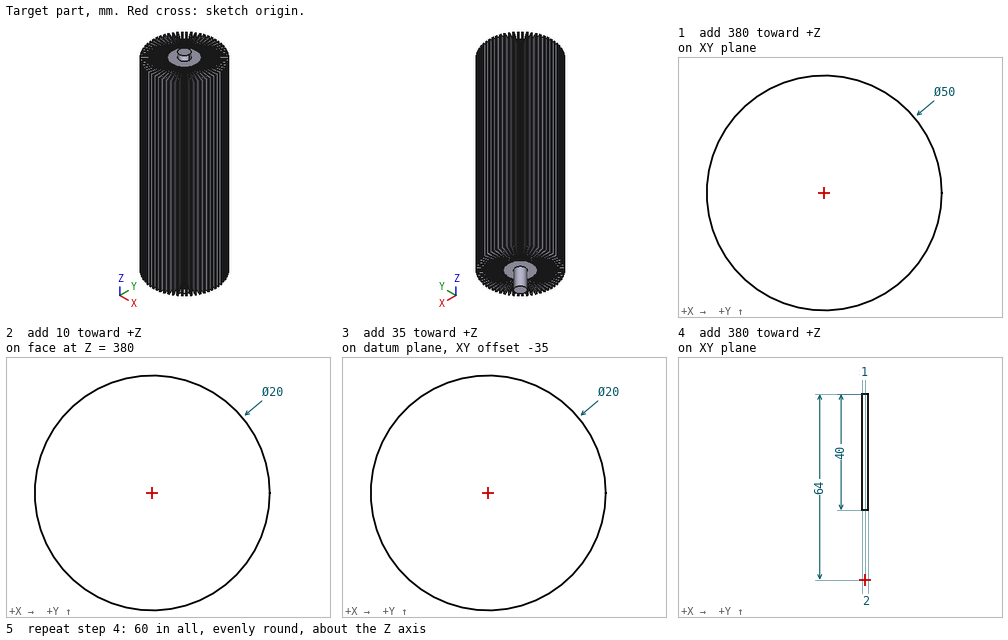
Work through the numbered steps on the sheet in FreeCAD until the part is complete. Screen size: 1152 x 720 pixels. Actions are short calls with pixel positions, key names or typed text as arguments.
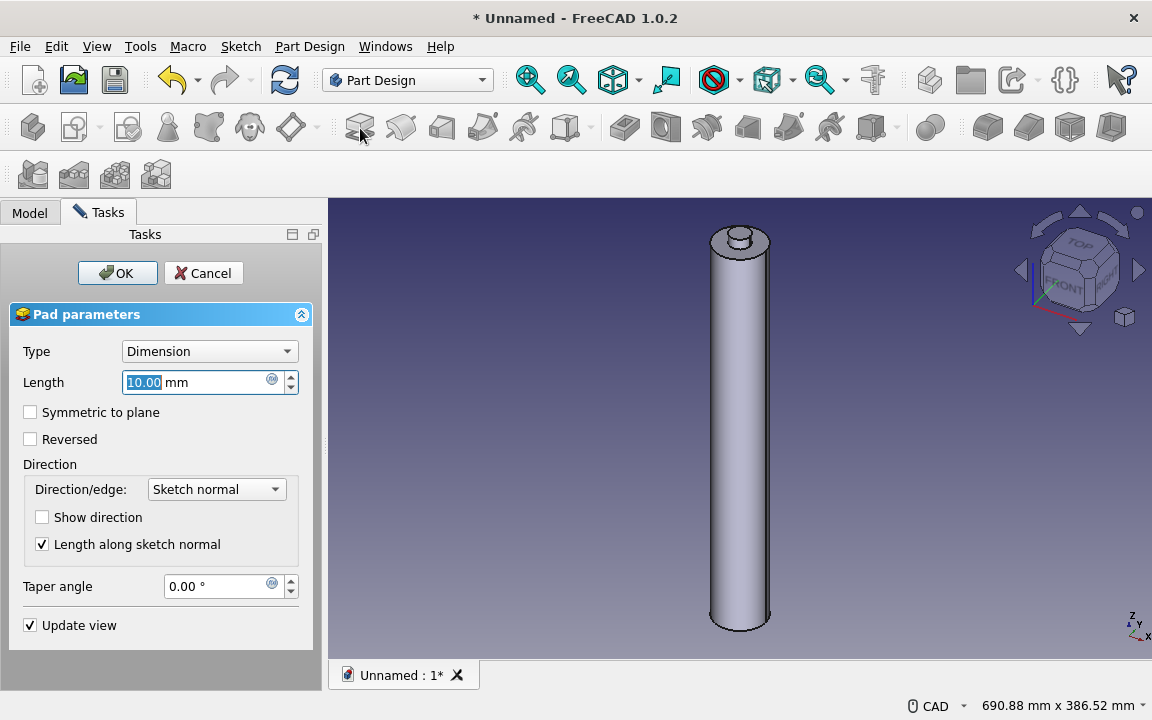
text(10)
key(Tab)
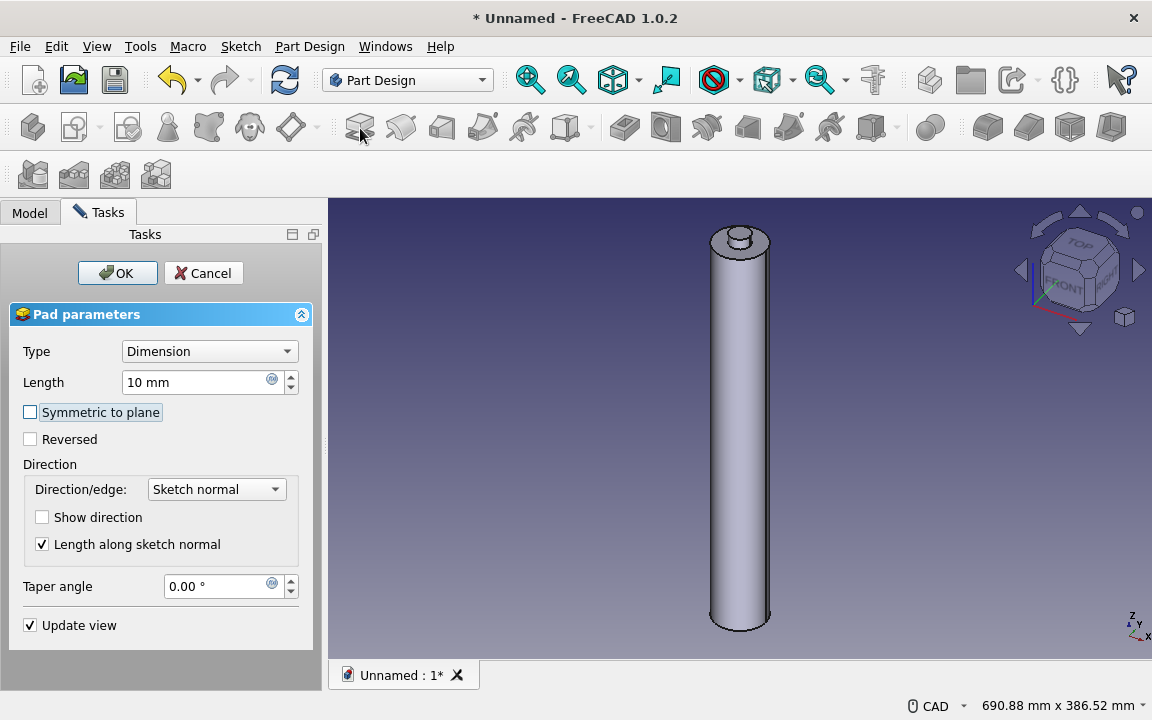
click(118, 273)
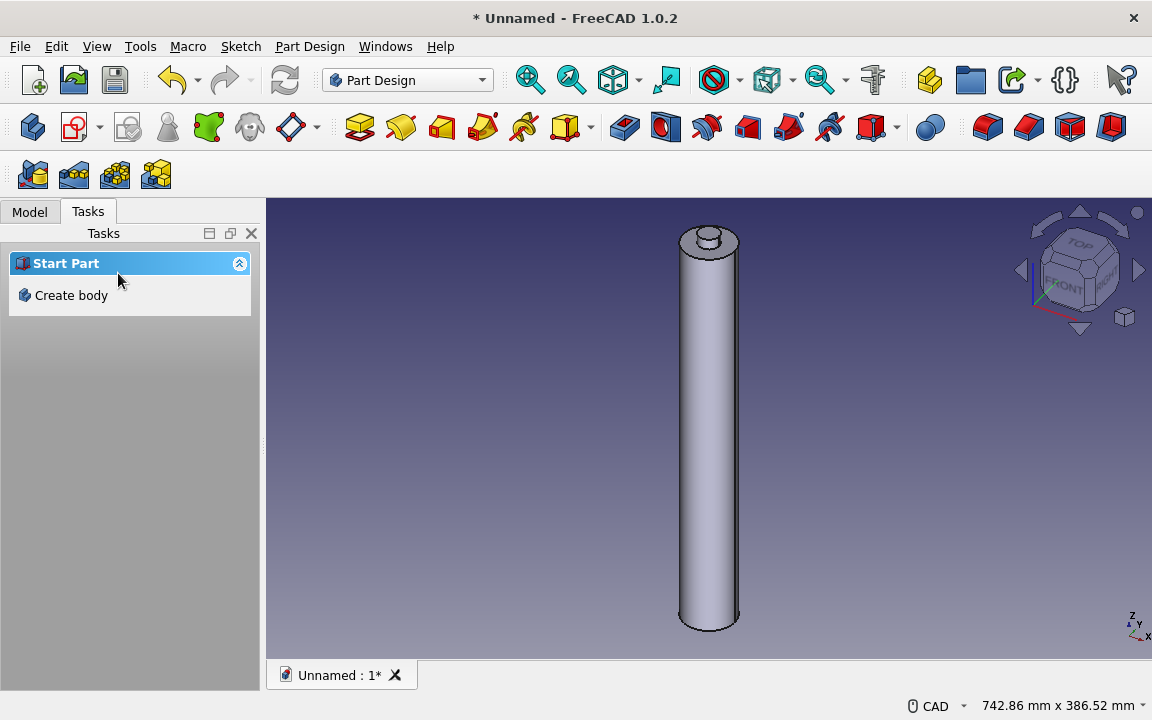
click(30, 212)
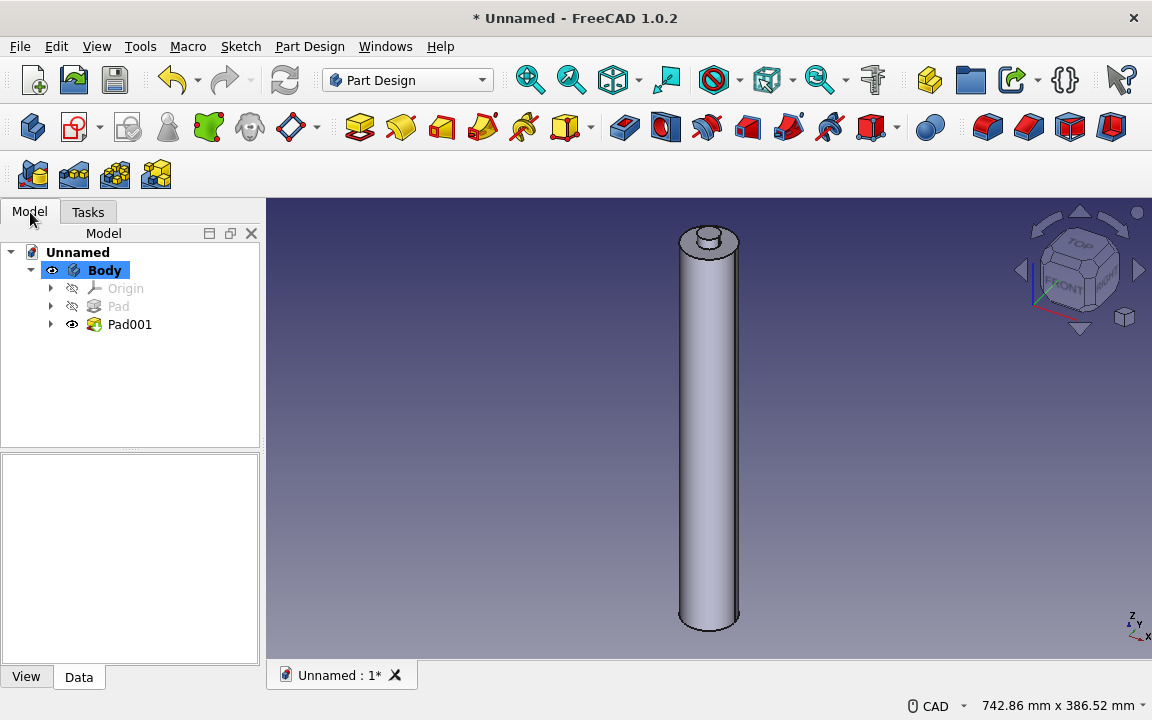
click(51, 288)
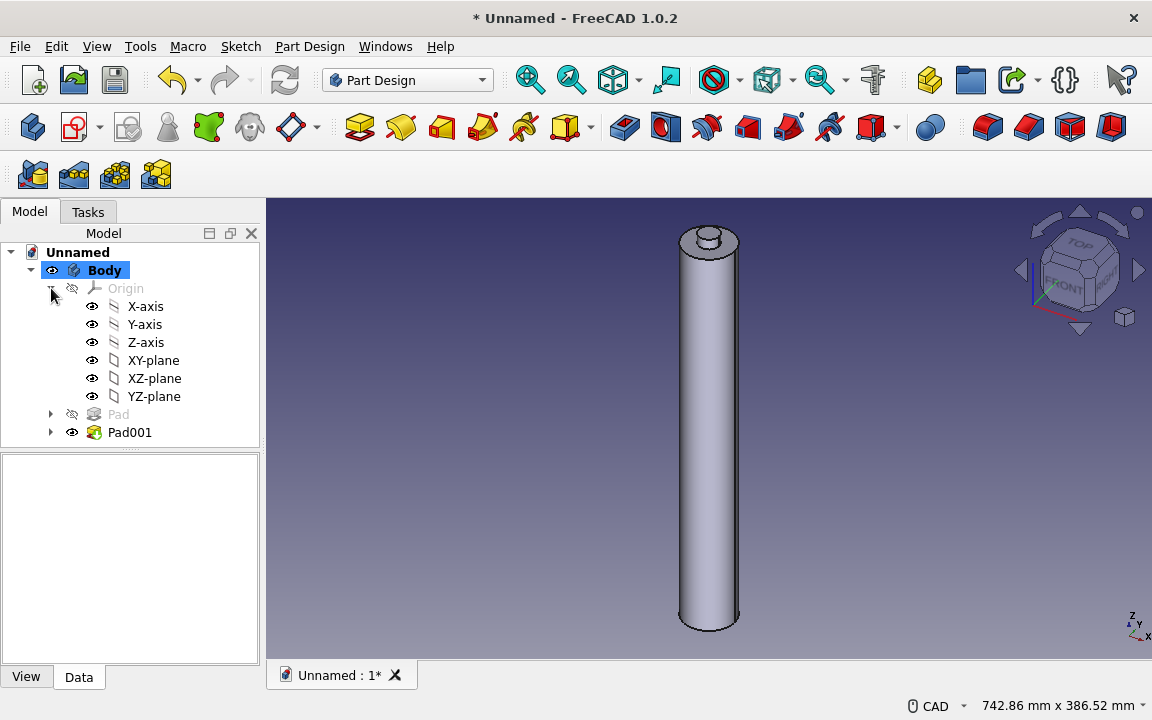
click(137, 360)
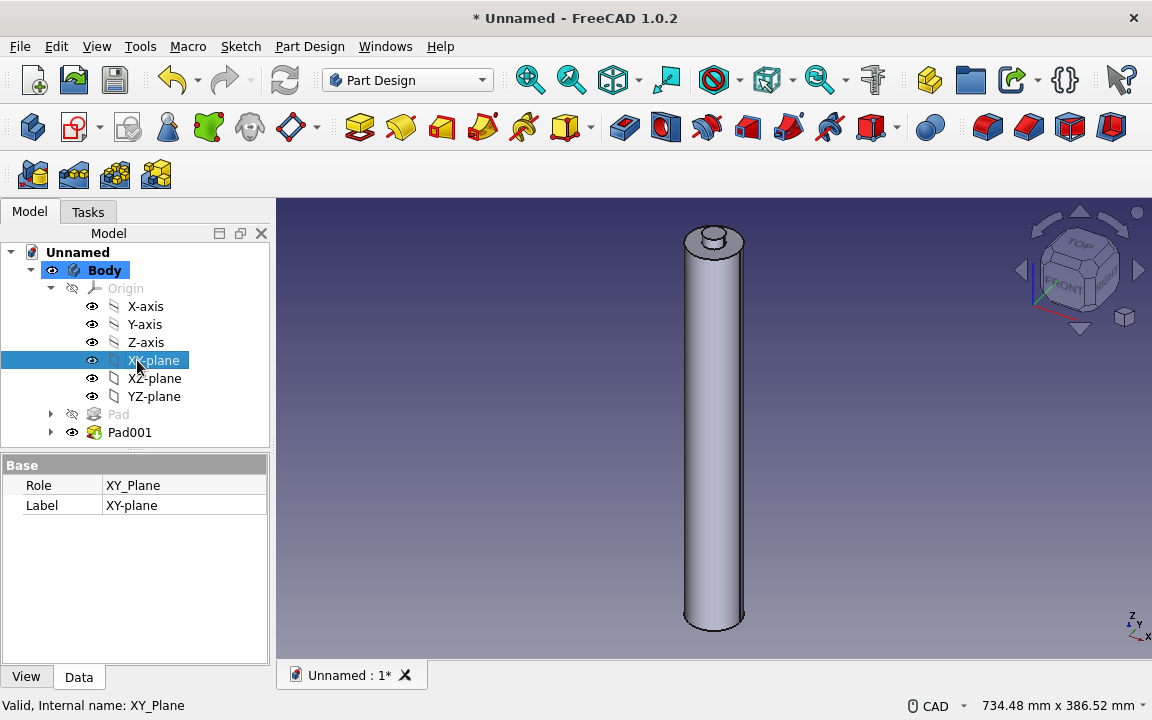
click(290, 128)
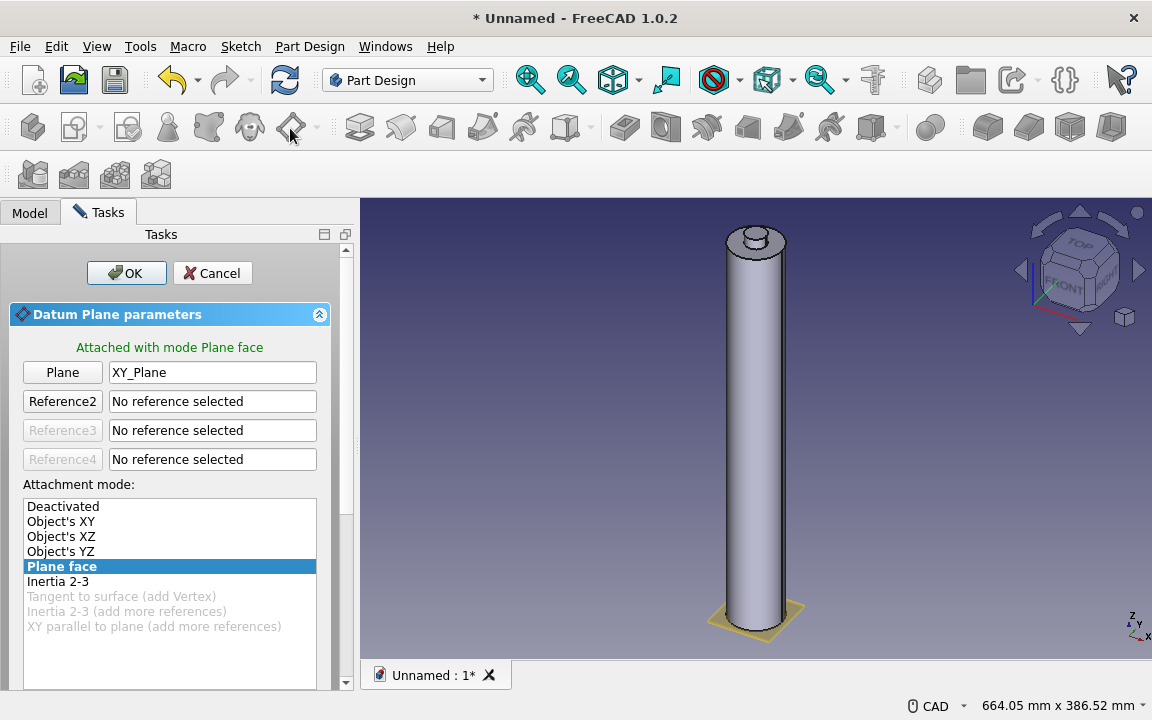
scroll(346, 467, down, 4)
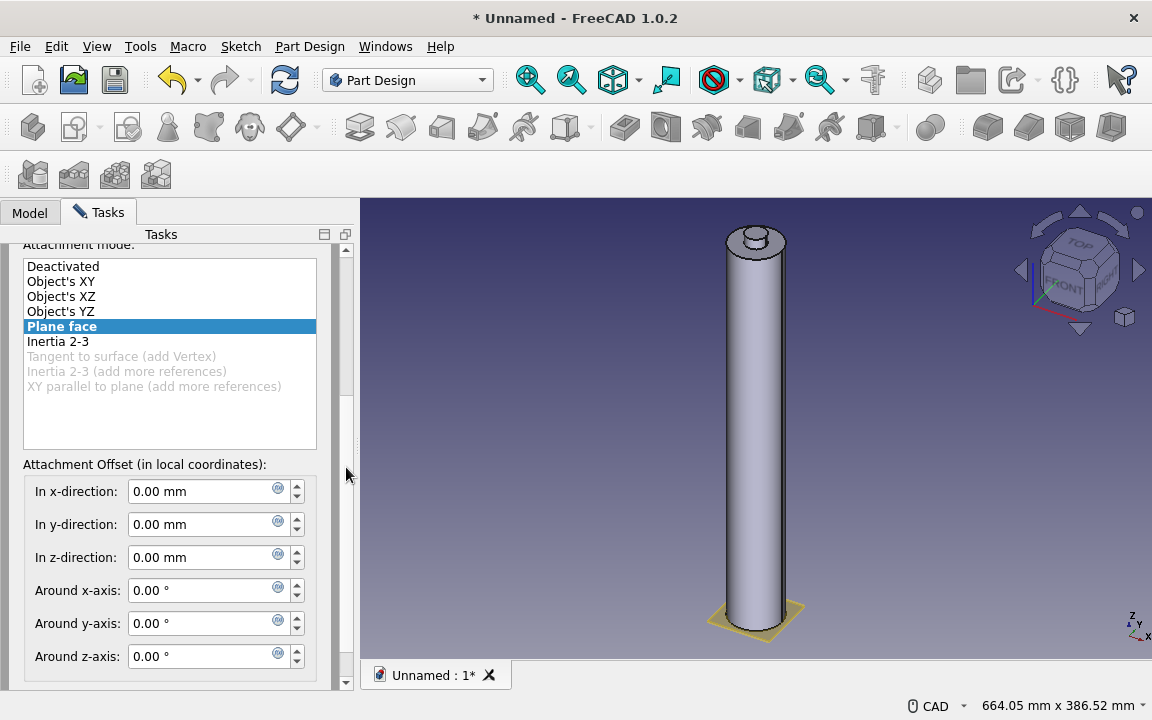
triple_click(210, 558)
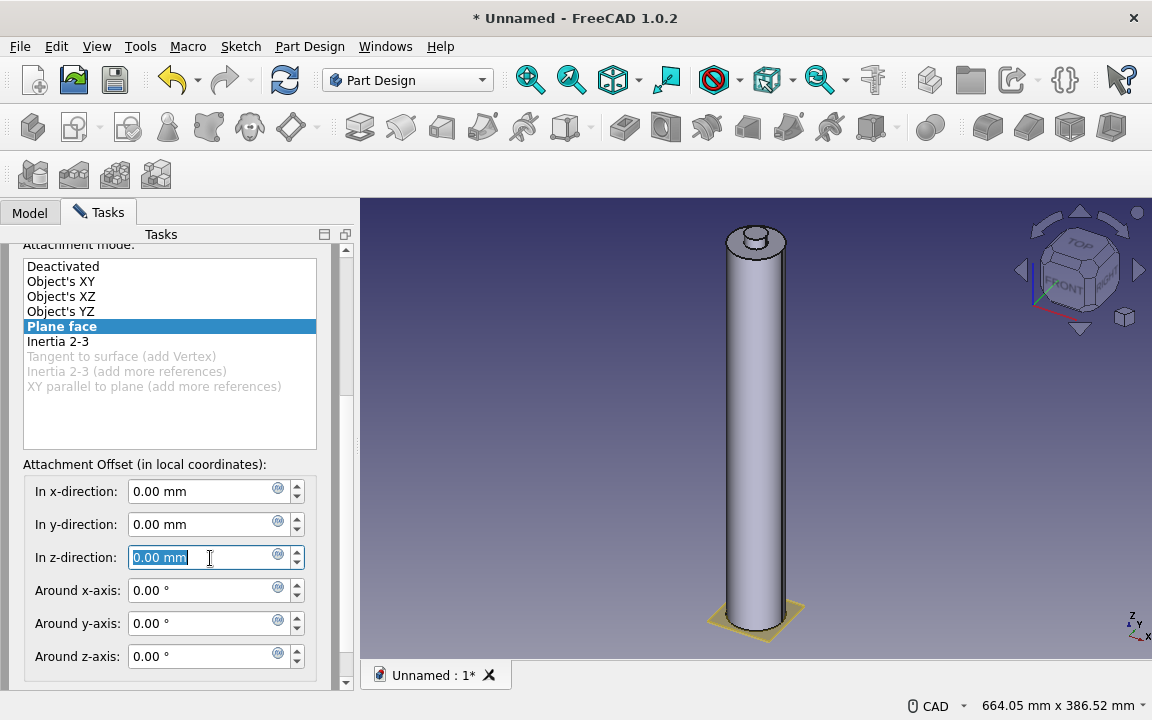
text(-35)
key(Tab)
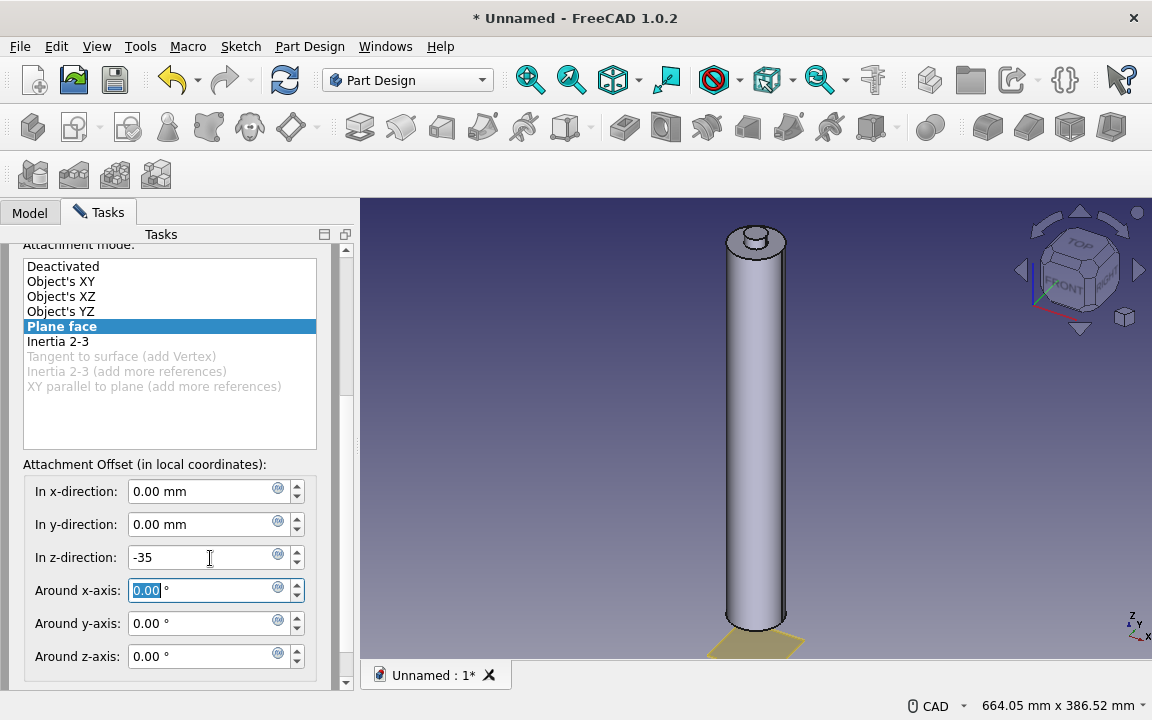
scroll(346, 467, up, 5)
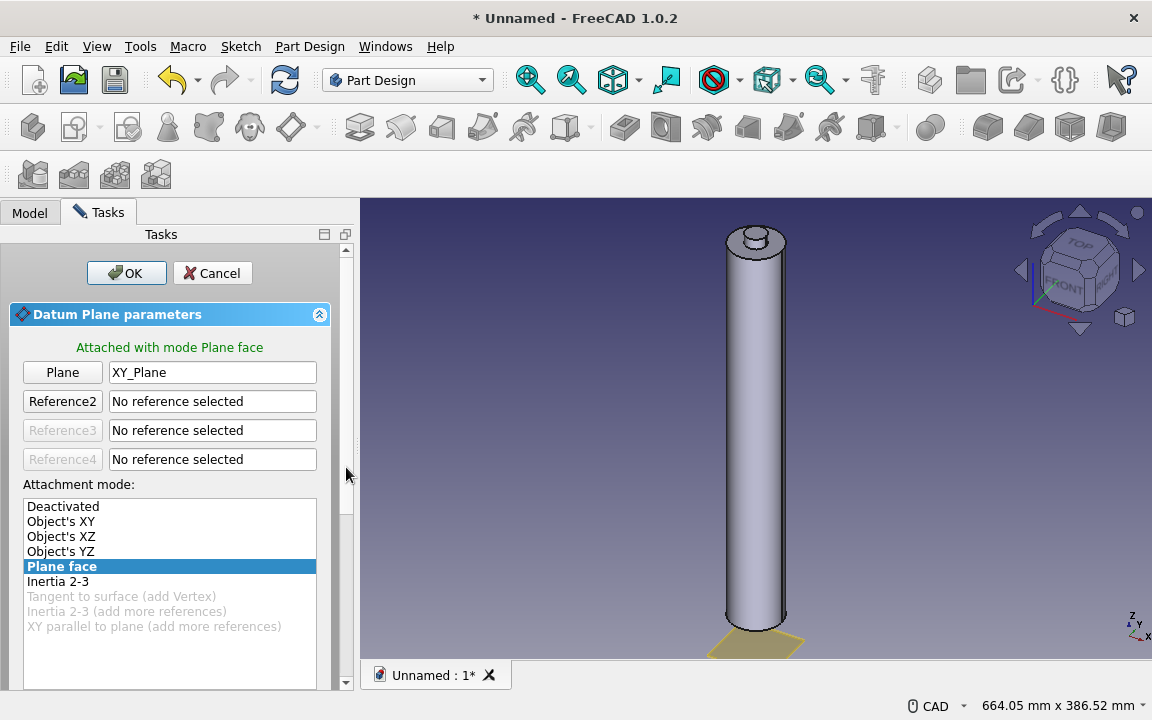
click(127, 273)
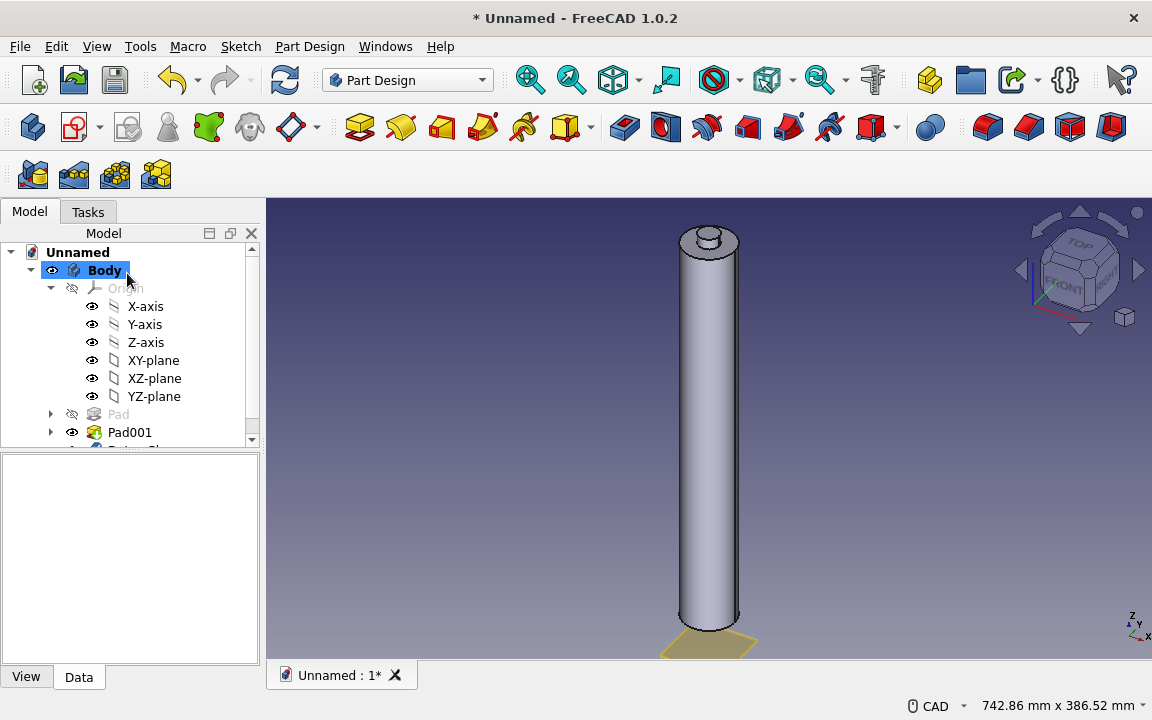
scroll(101, 338, down, 3)